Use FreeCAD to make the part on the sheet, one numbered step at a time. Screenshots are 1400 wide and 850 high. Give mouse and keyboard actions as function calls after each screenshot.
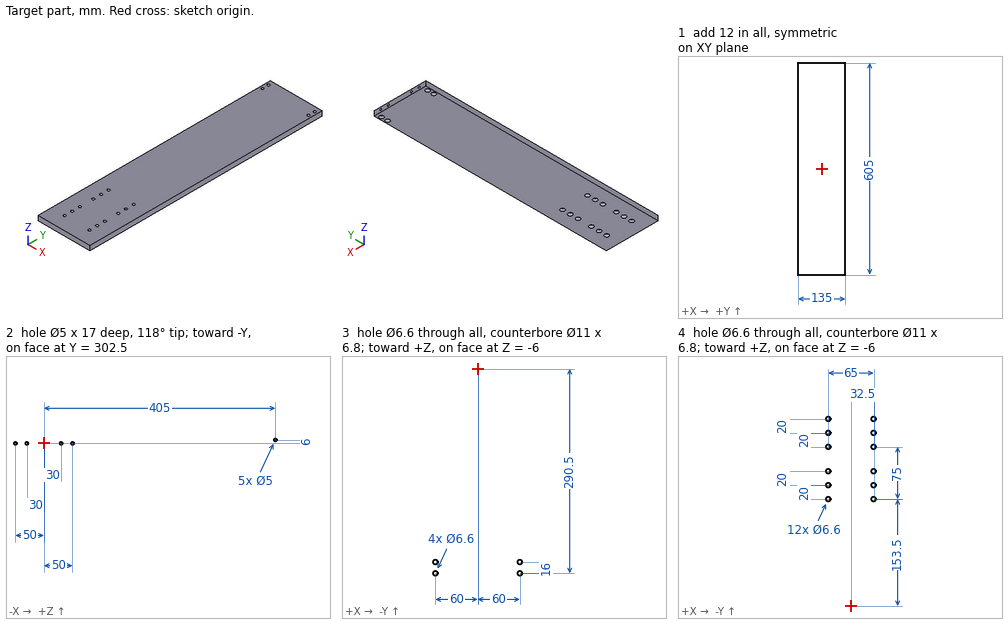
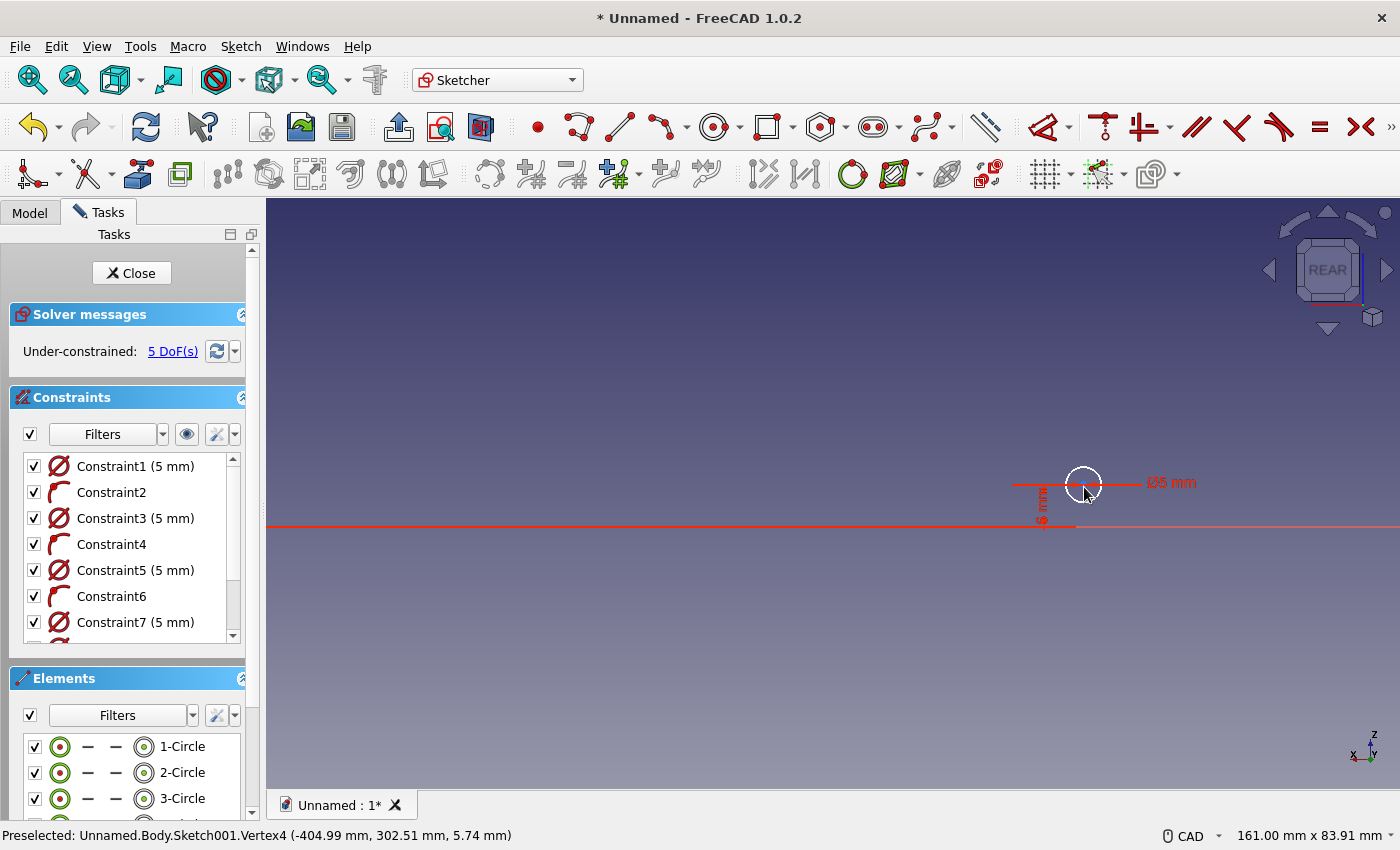
scroll(1089, 490, down, 8)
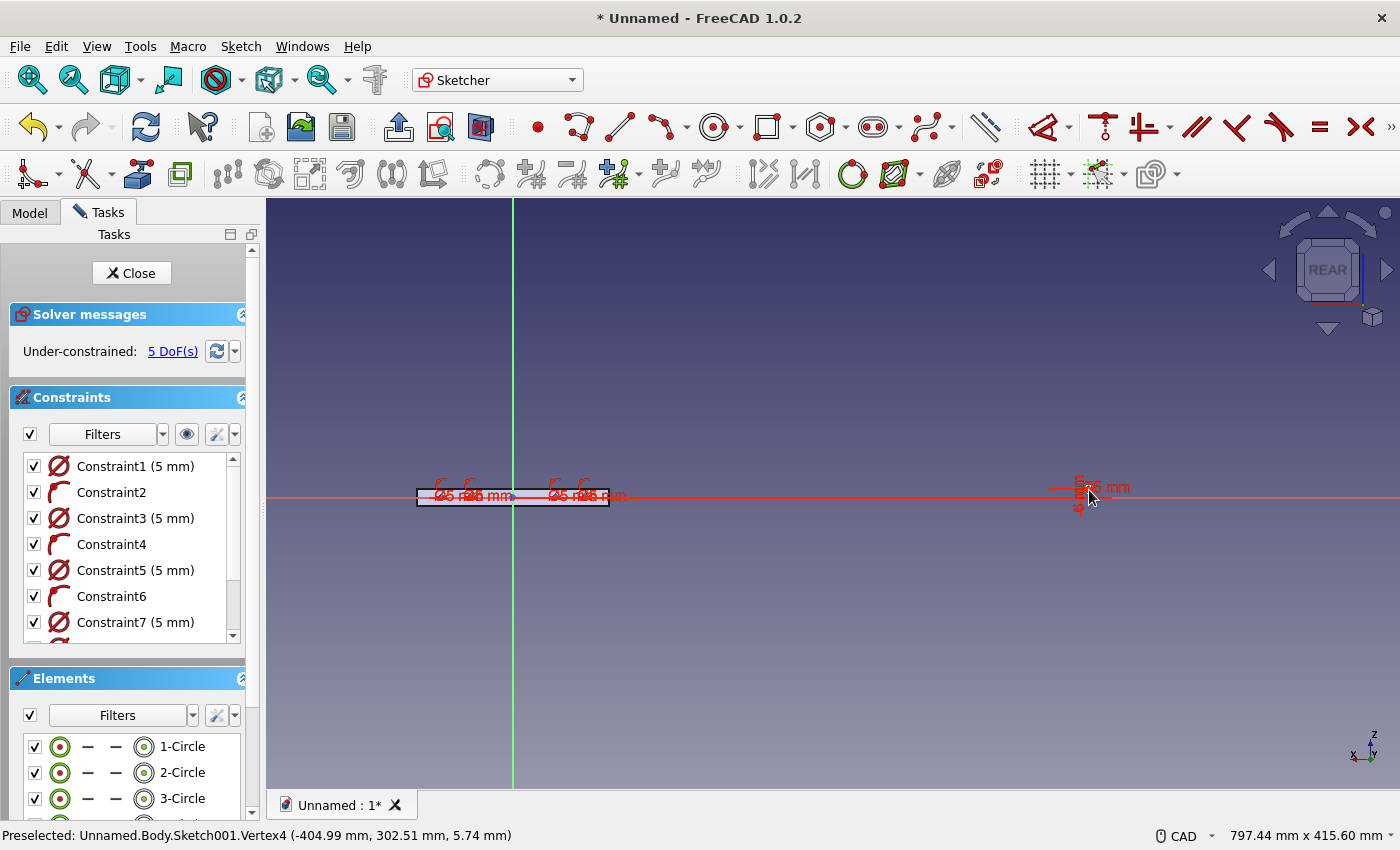
click(441, 498)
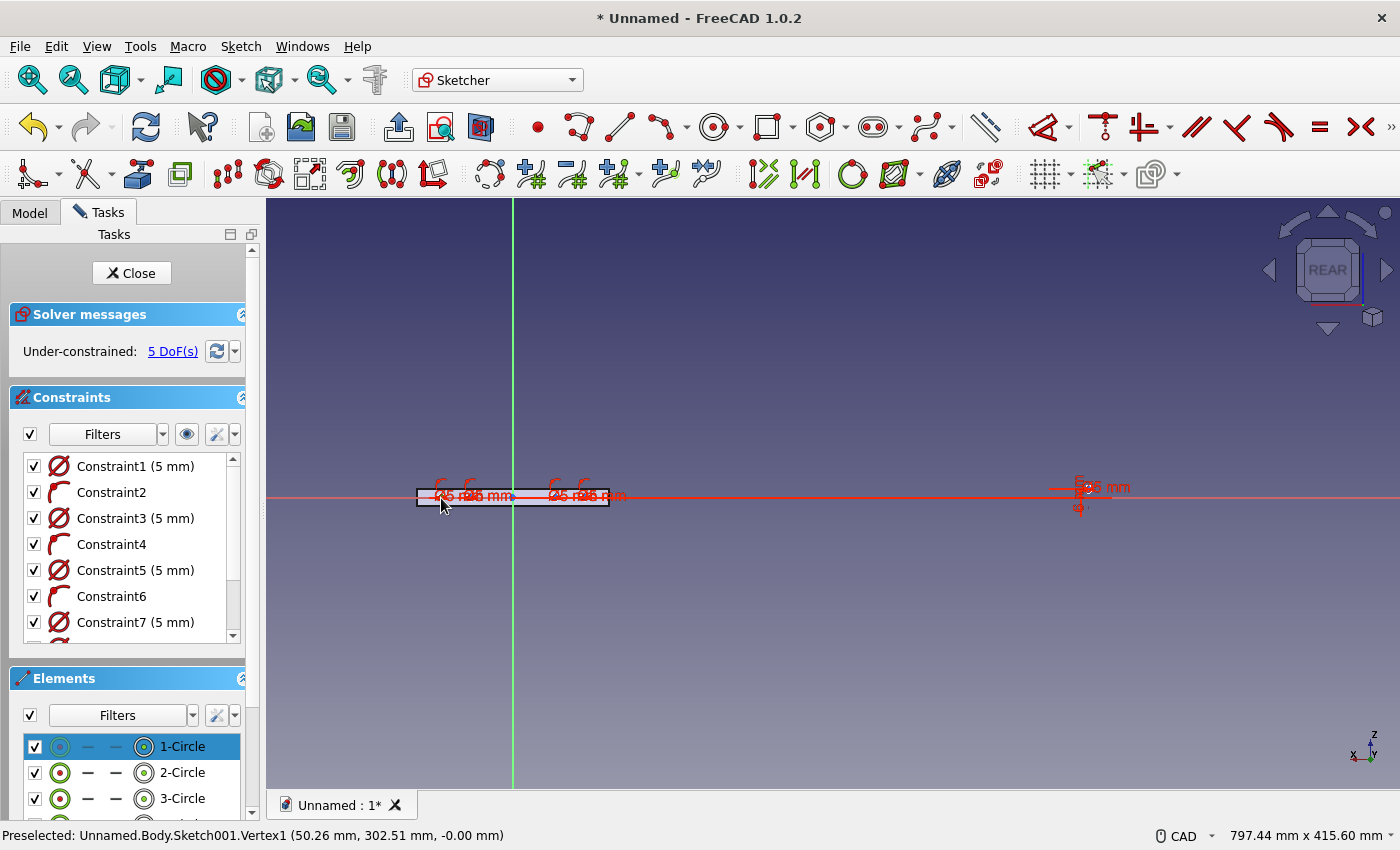
key(l)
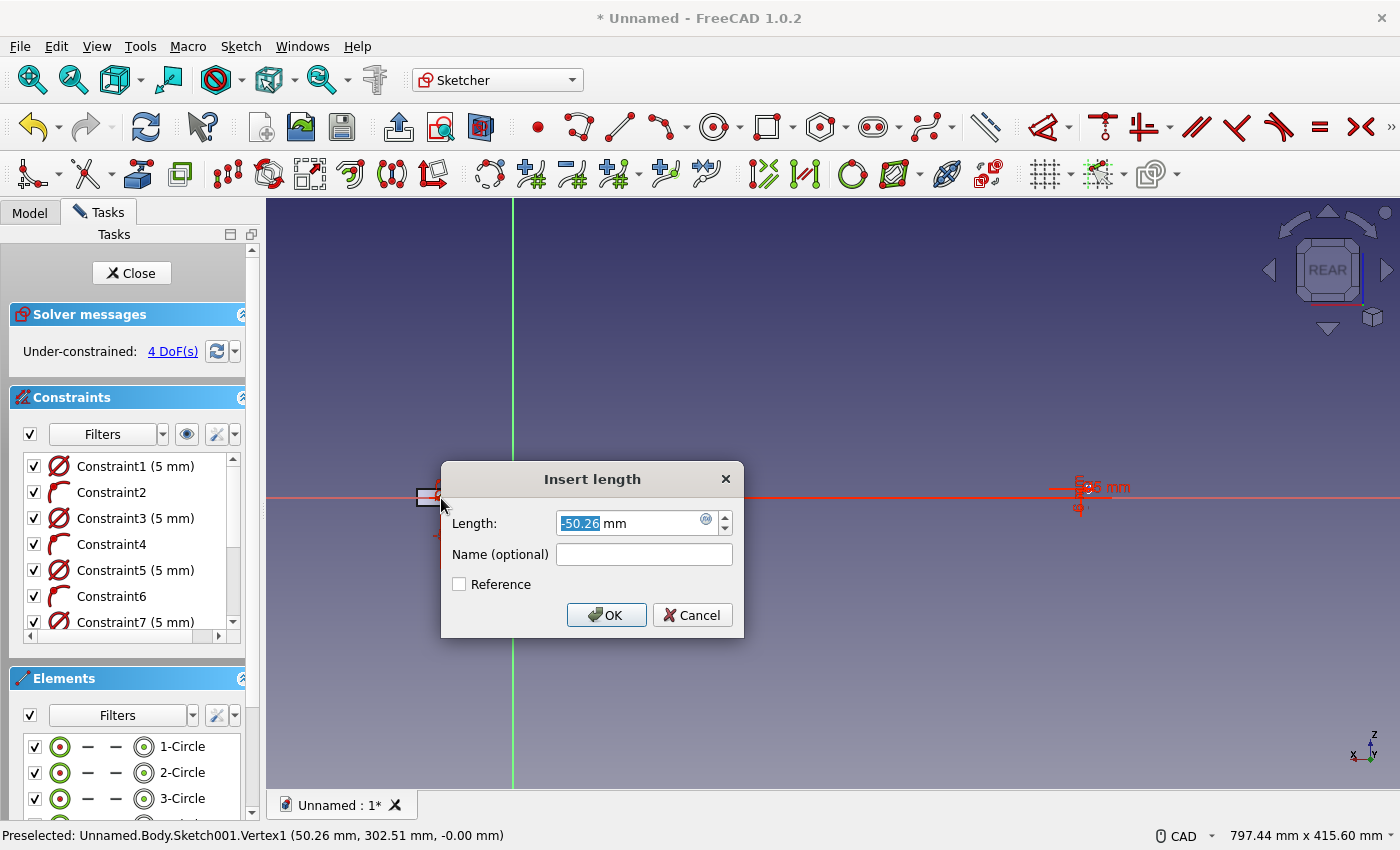
text(-50)
key(Return)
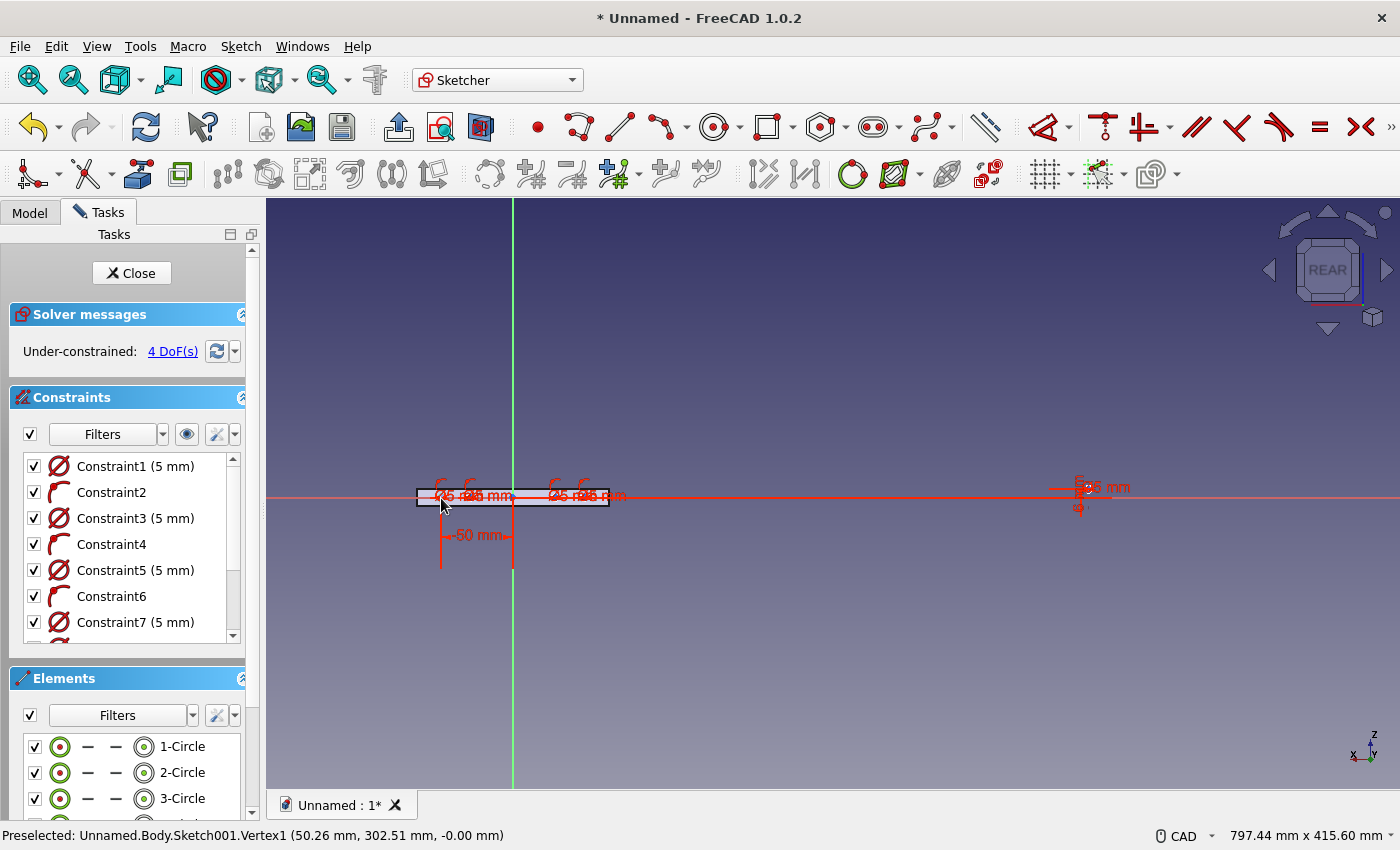
click(555, 498)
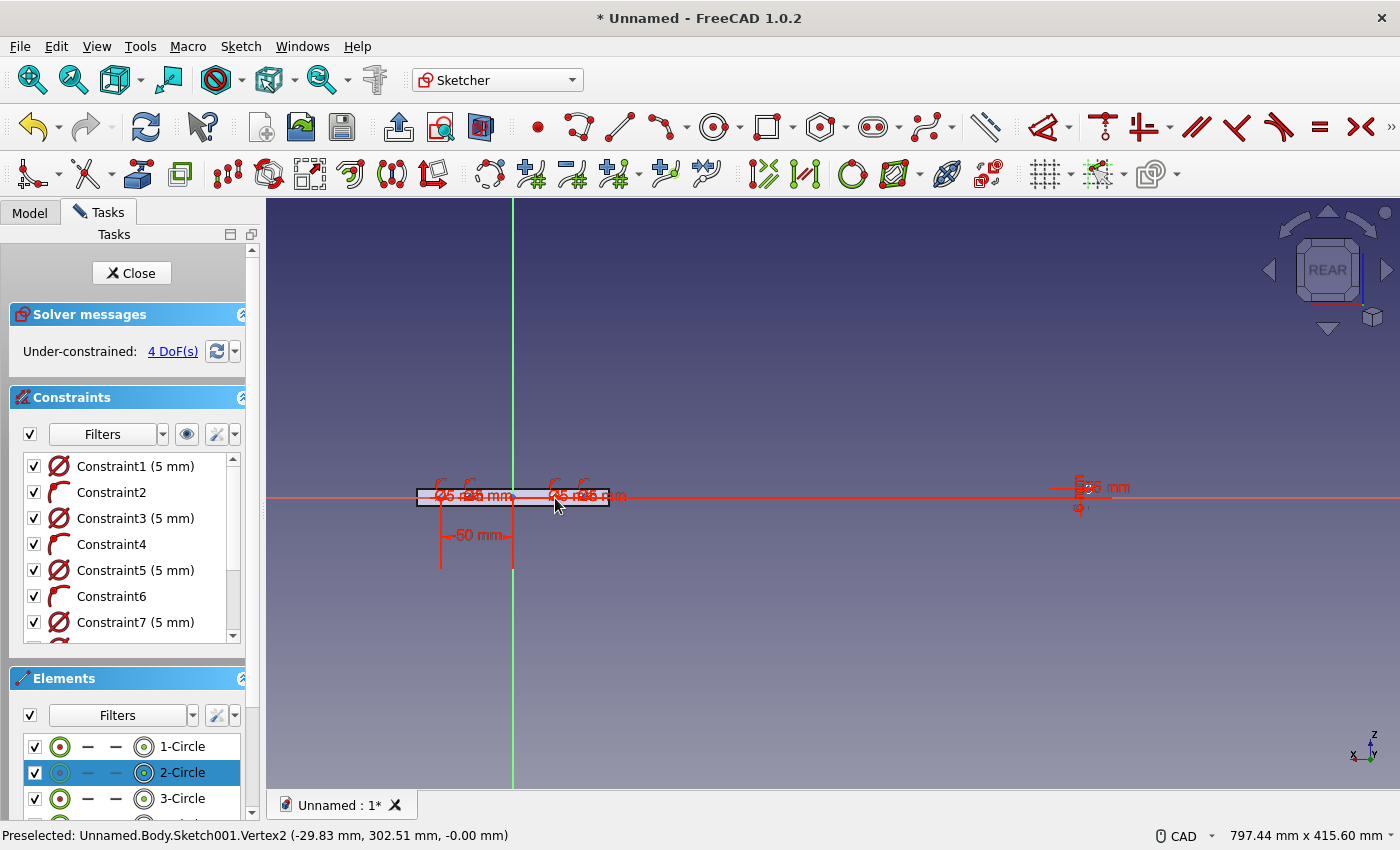
key(l)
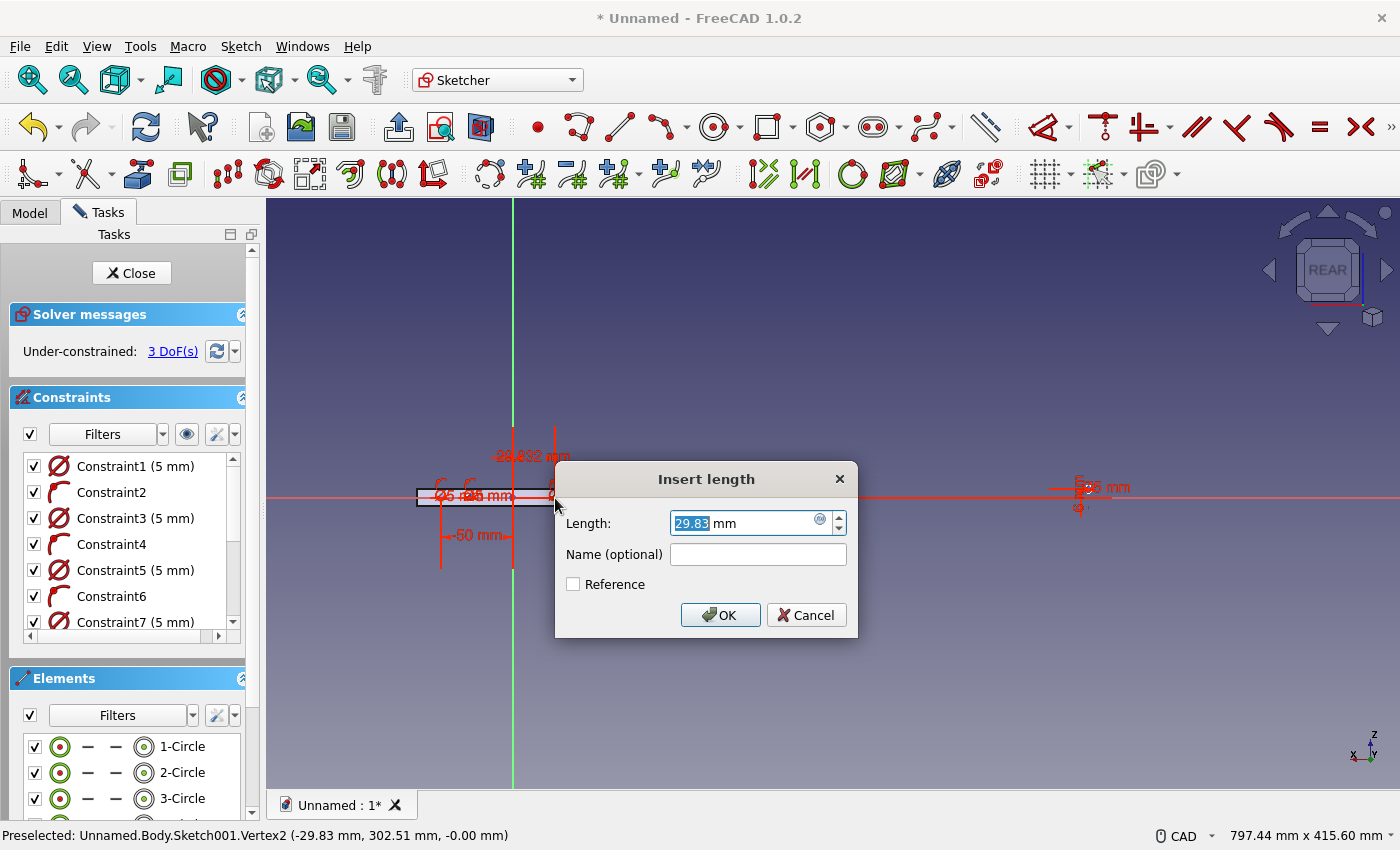
text(30)
key(Return)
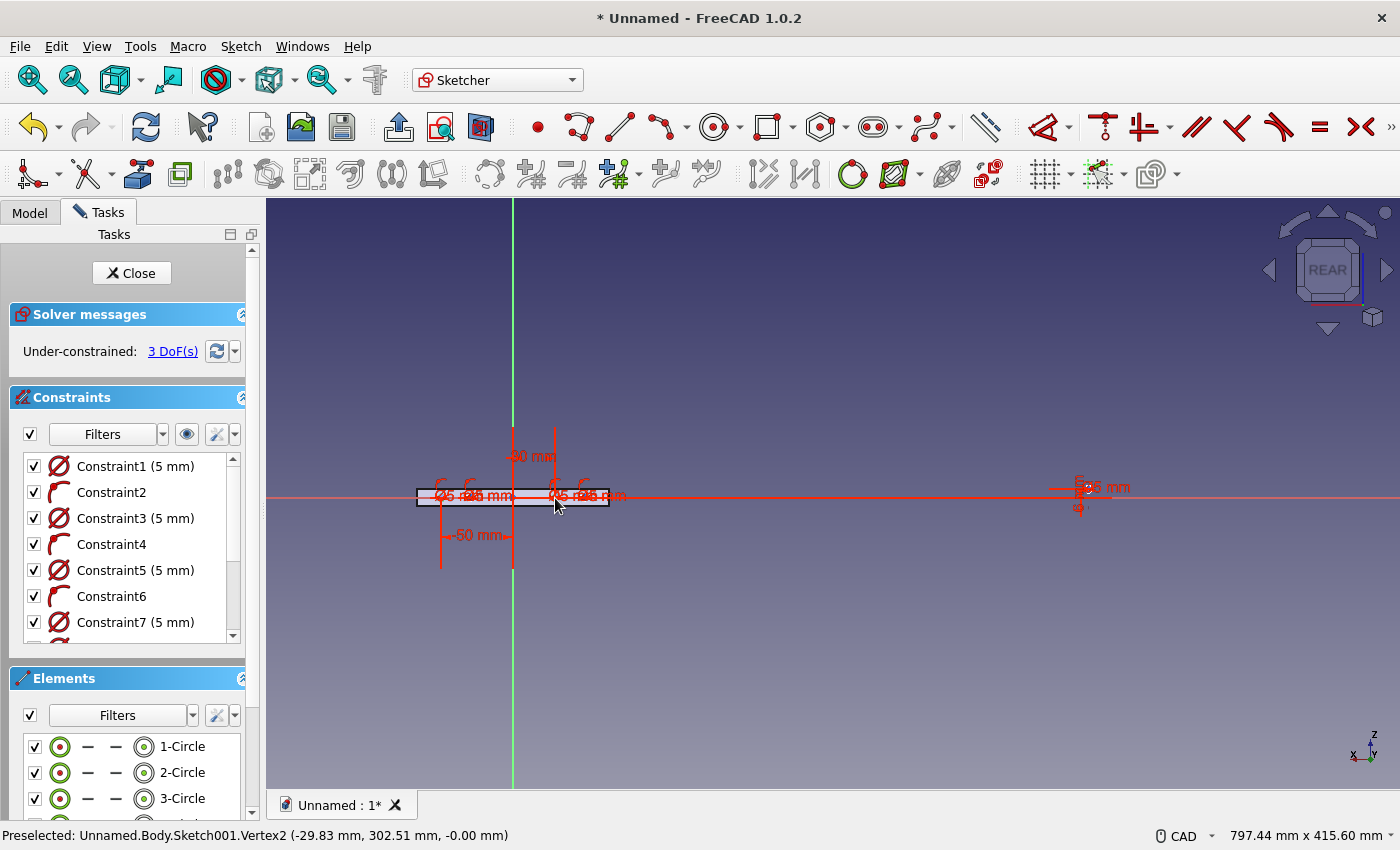
click(470, 498)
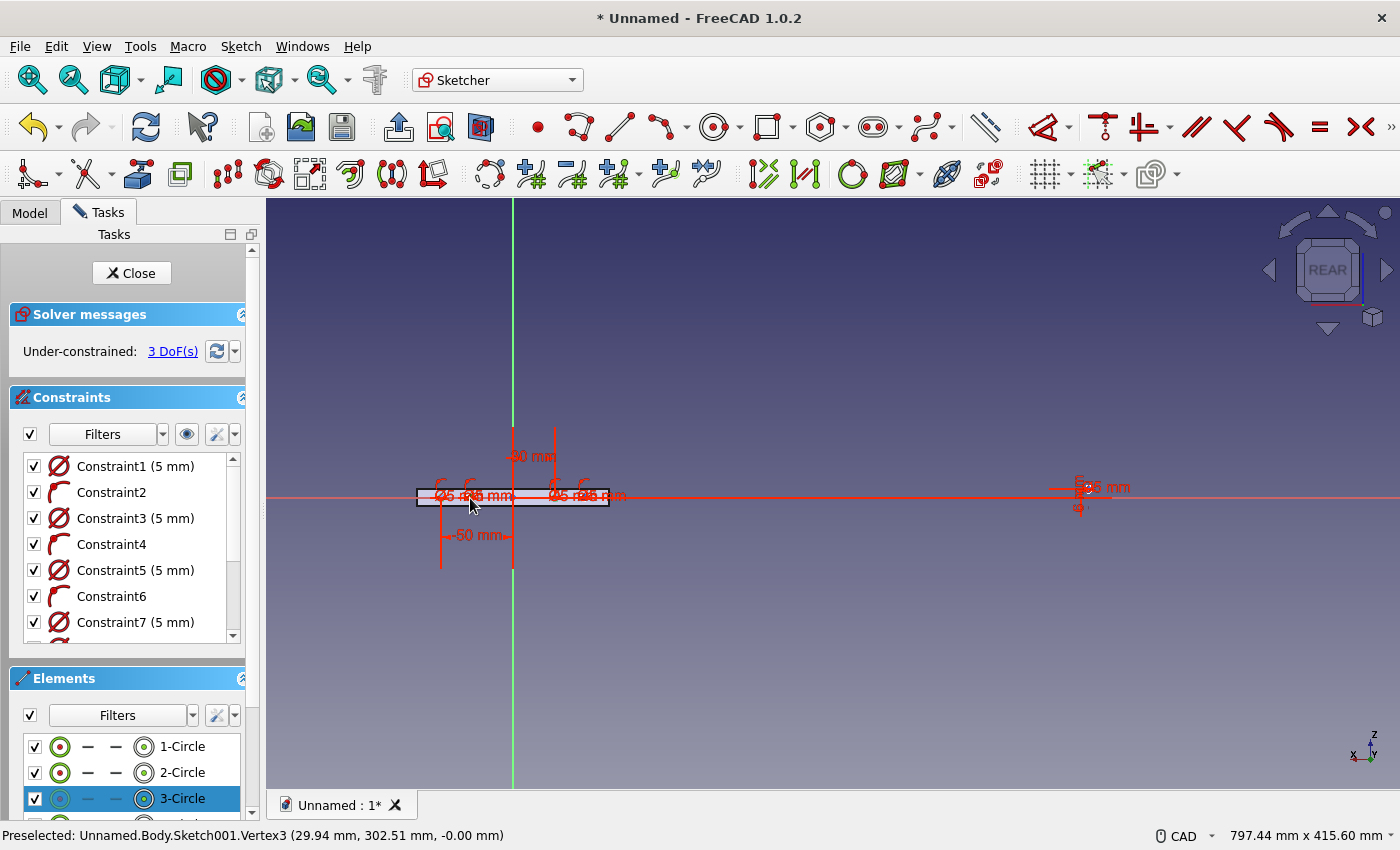
click(1068, 128)